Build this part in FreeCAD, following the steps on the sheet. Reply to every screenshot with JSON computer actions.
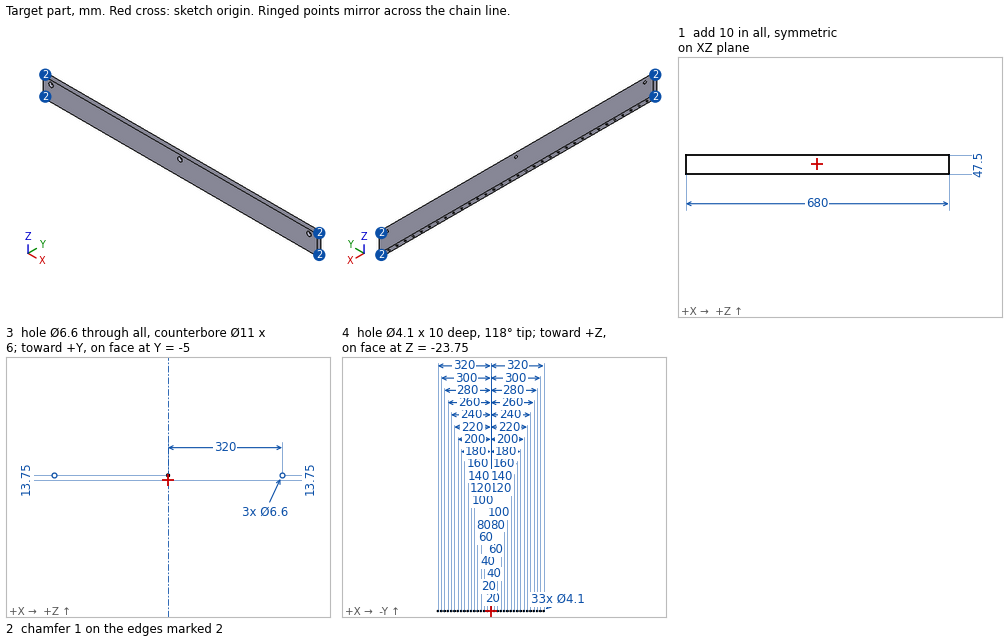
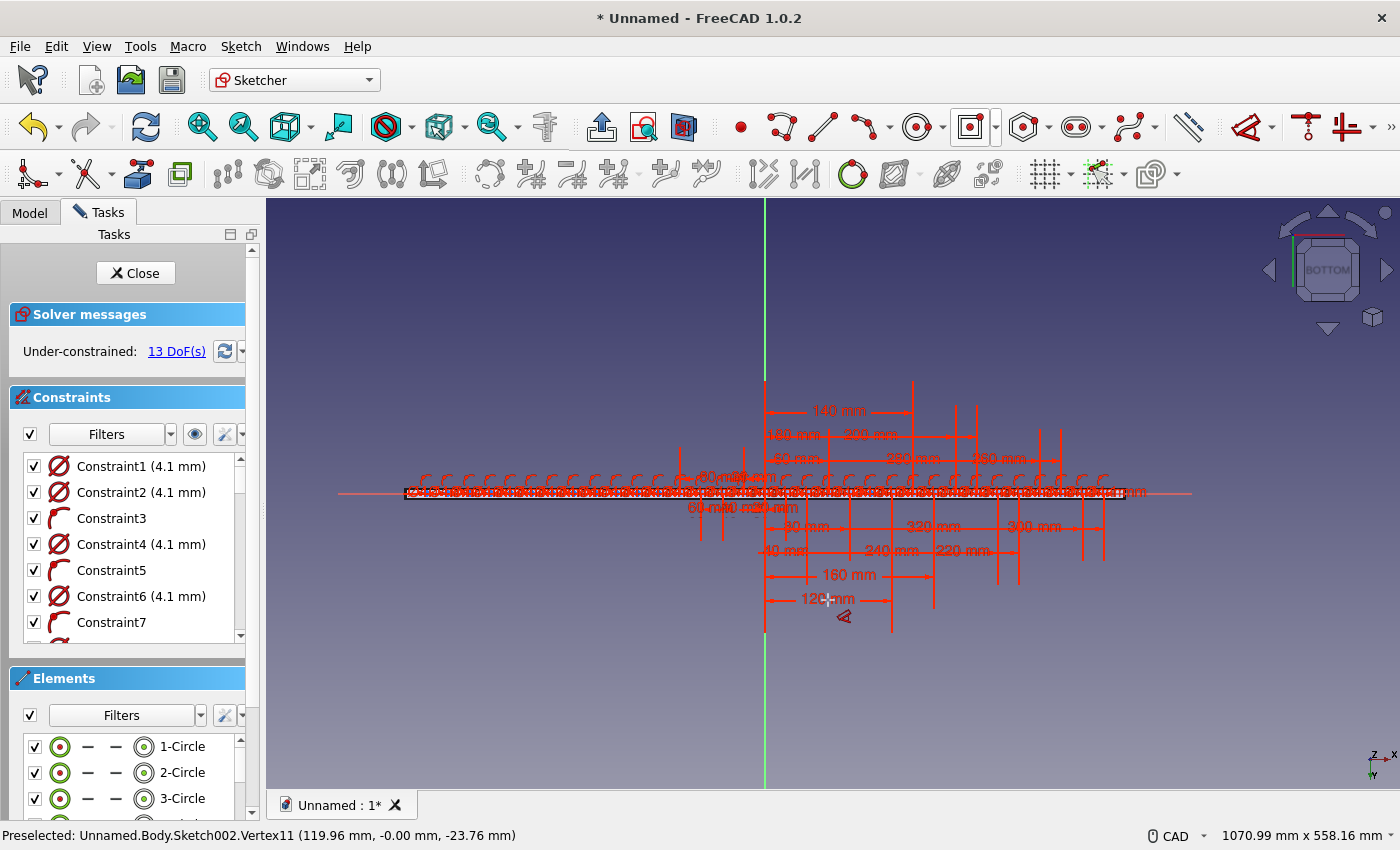
{"action": "left_click", "coordinate": [871, 494]}
{"action": "left_click", "coordinate": [818, 388]}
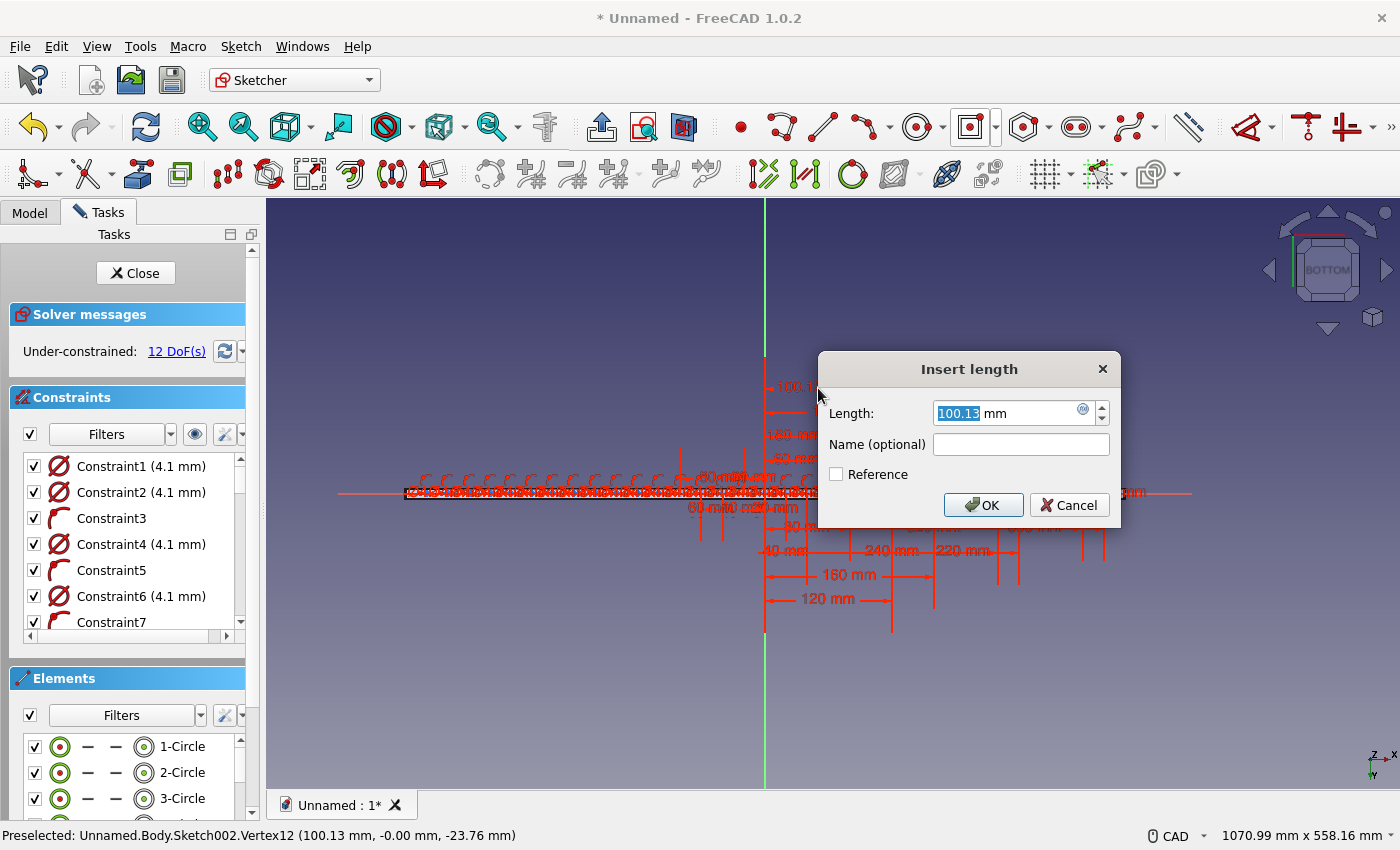
{"action": "type", "text": "100"}
{"action": "key", "text": "Return"}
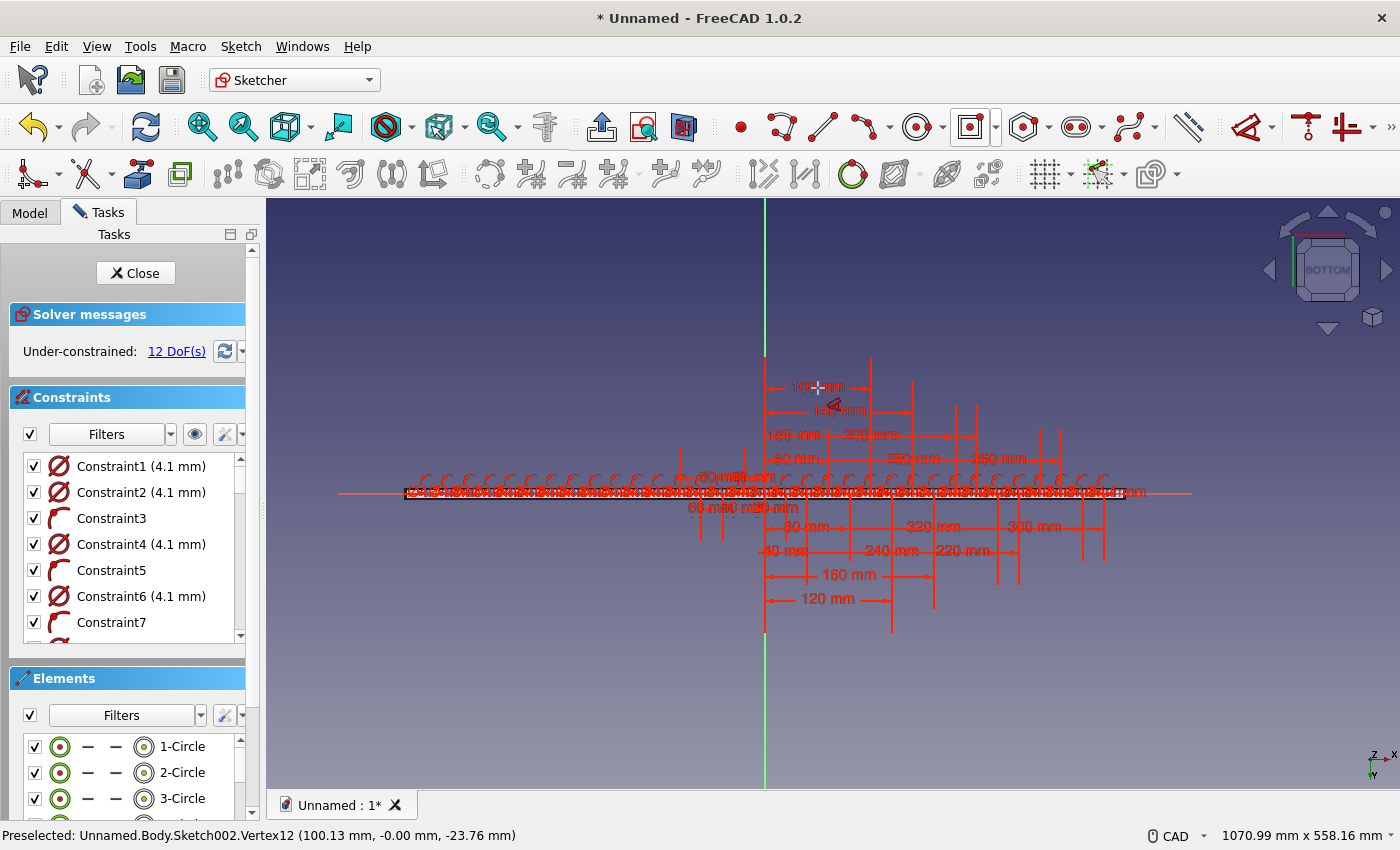
{"action": "left_click", "coordinate": [659, 494]}
{"action": "left_click", "coordinate": [712, 552]}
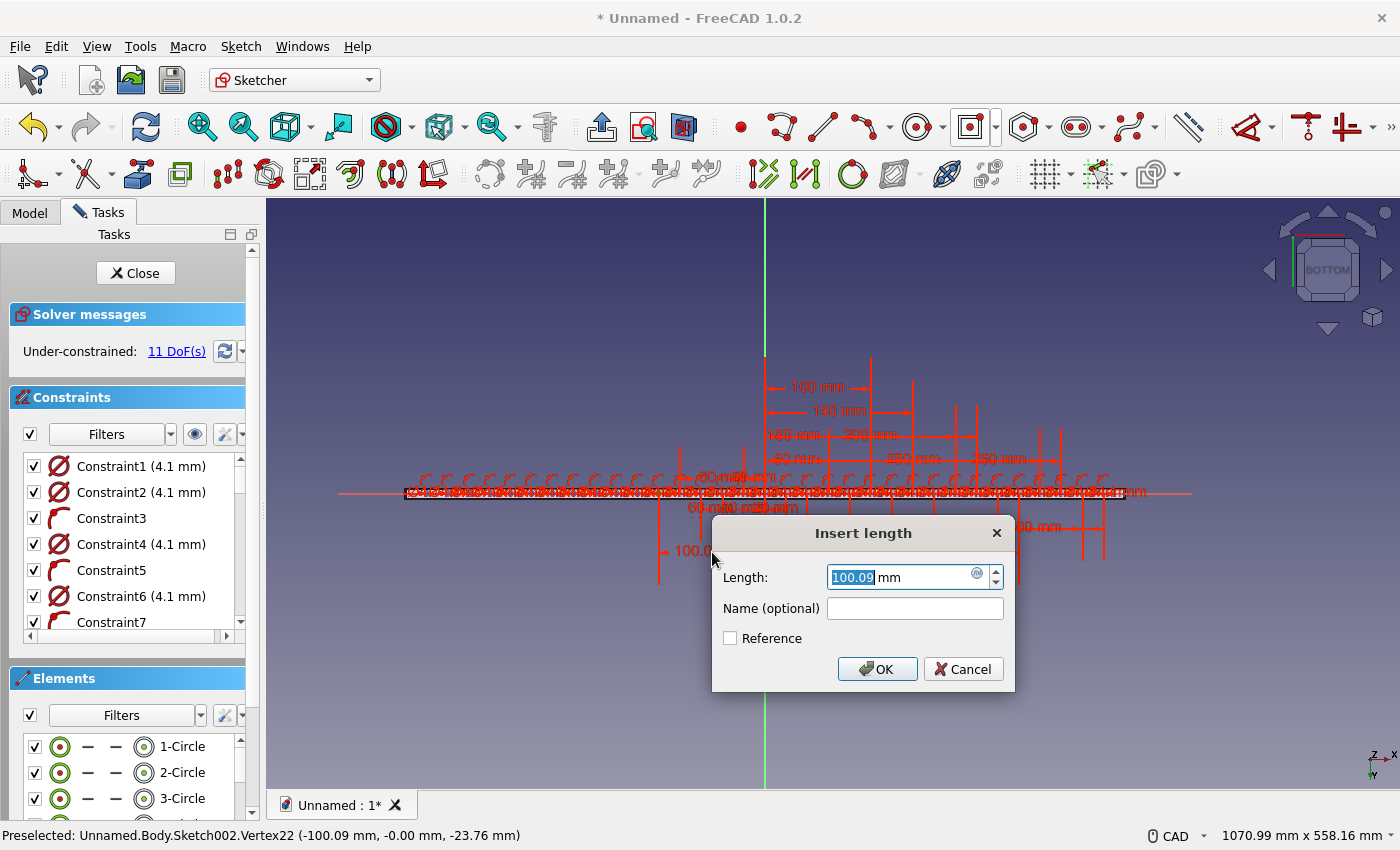
{"action": "type", "text": "100"}
{"action": "key", "text": "Return"}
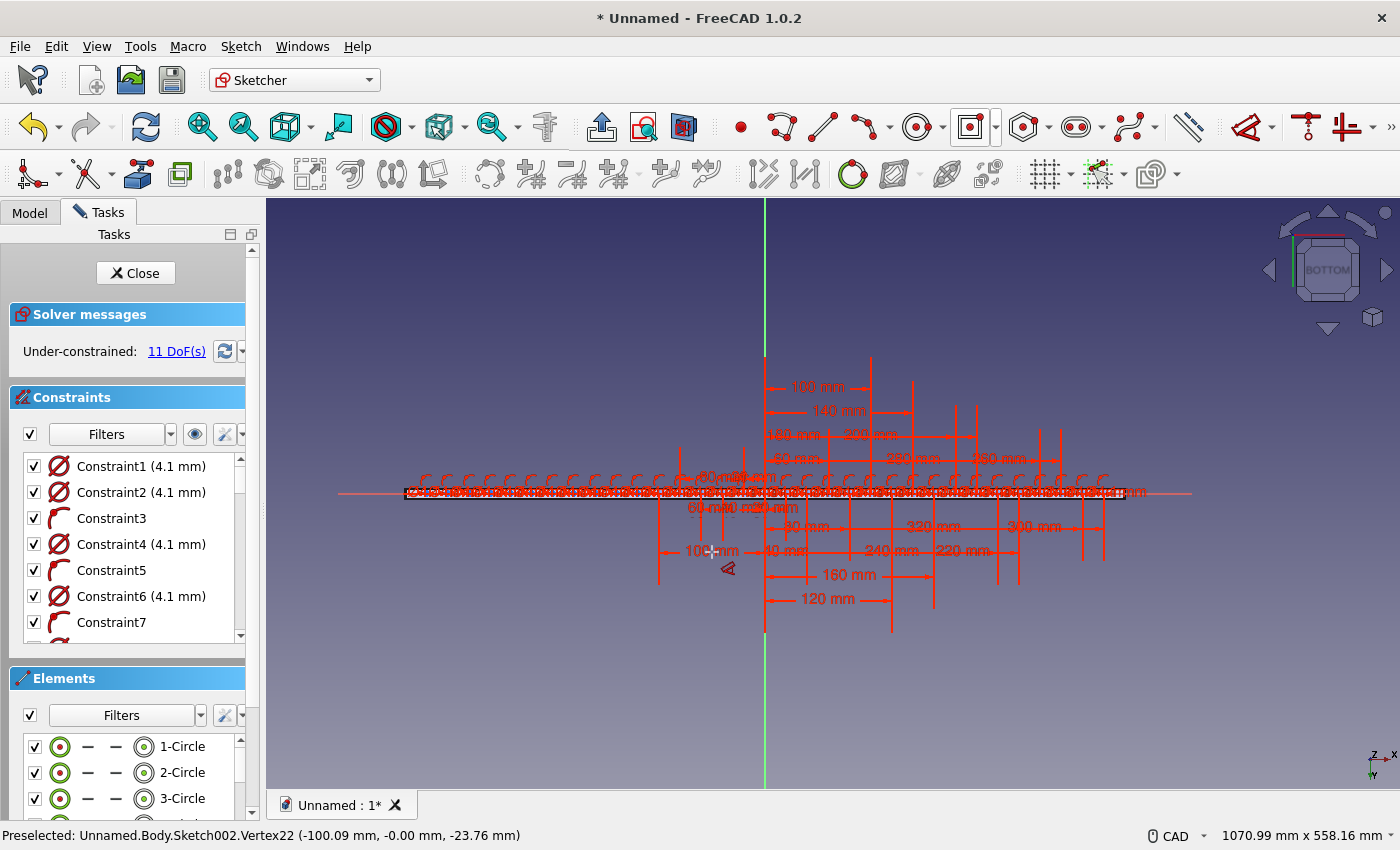
{"action": "left_click", "coordinate": [638, 494]}
{"action": "left_click", "coordinate": [701, 436]}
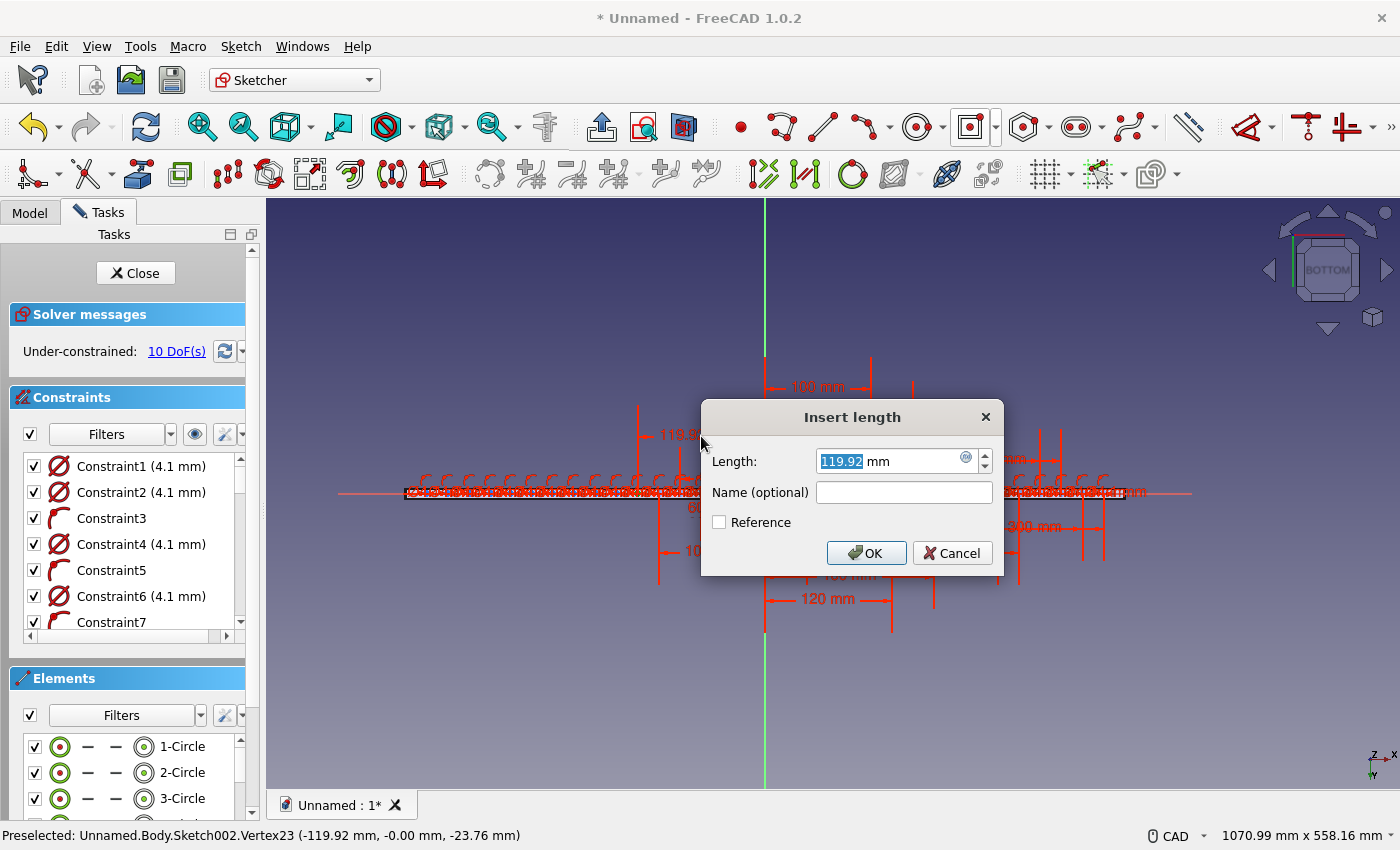
{"action": "type", "text": "120"}
{"action": "key", "text": "Return"}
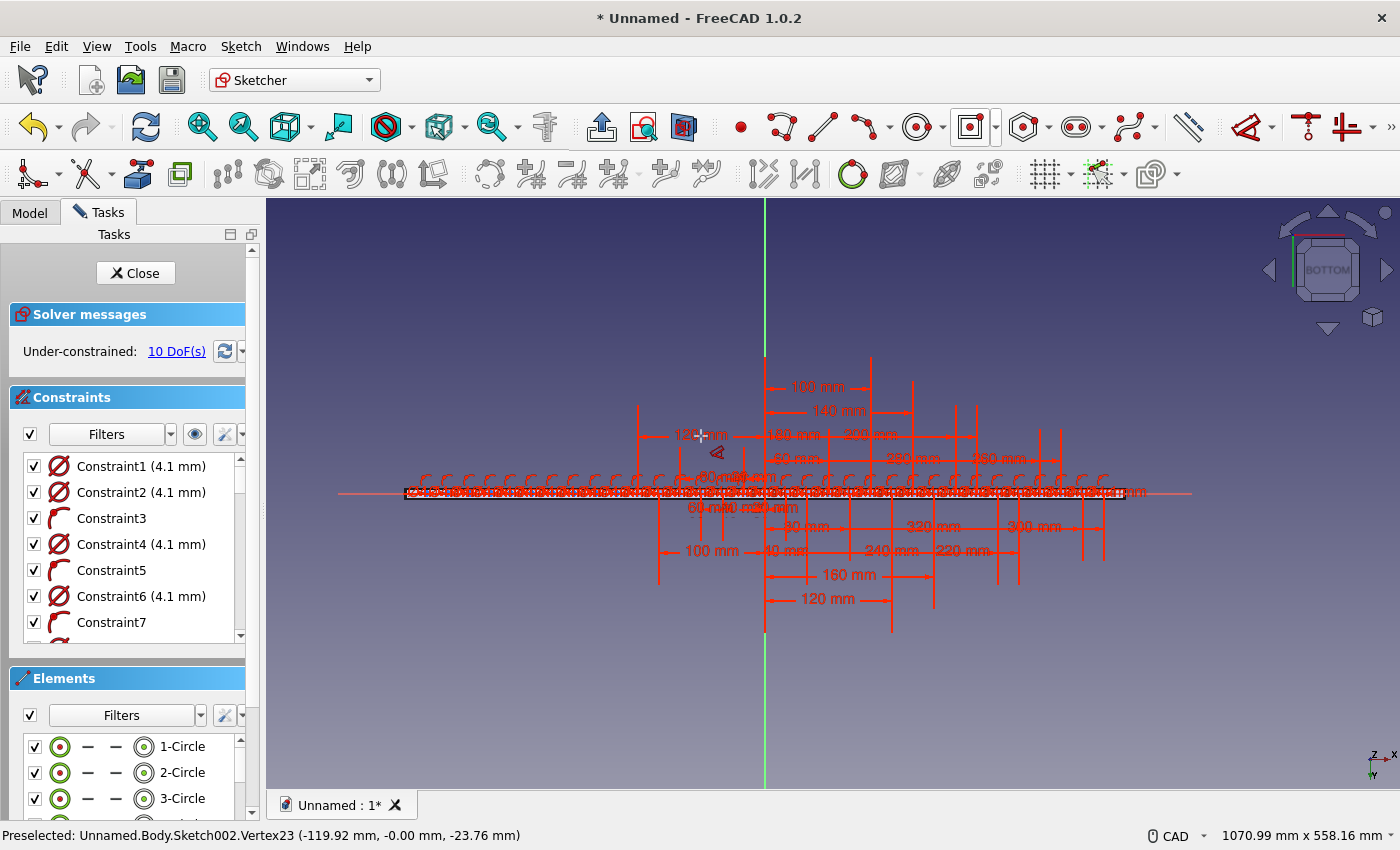
{"action": "left_click", "coordinate": [617, 494]}
{"action": "left_click", "coordinate": [639, 528]}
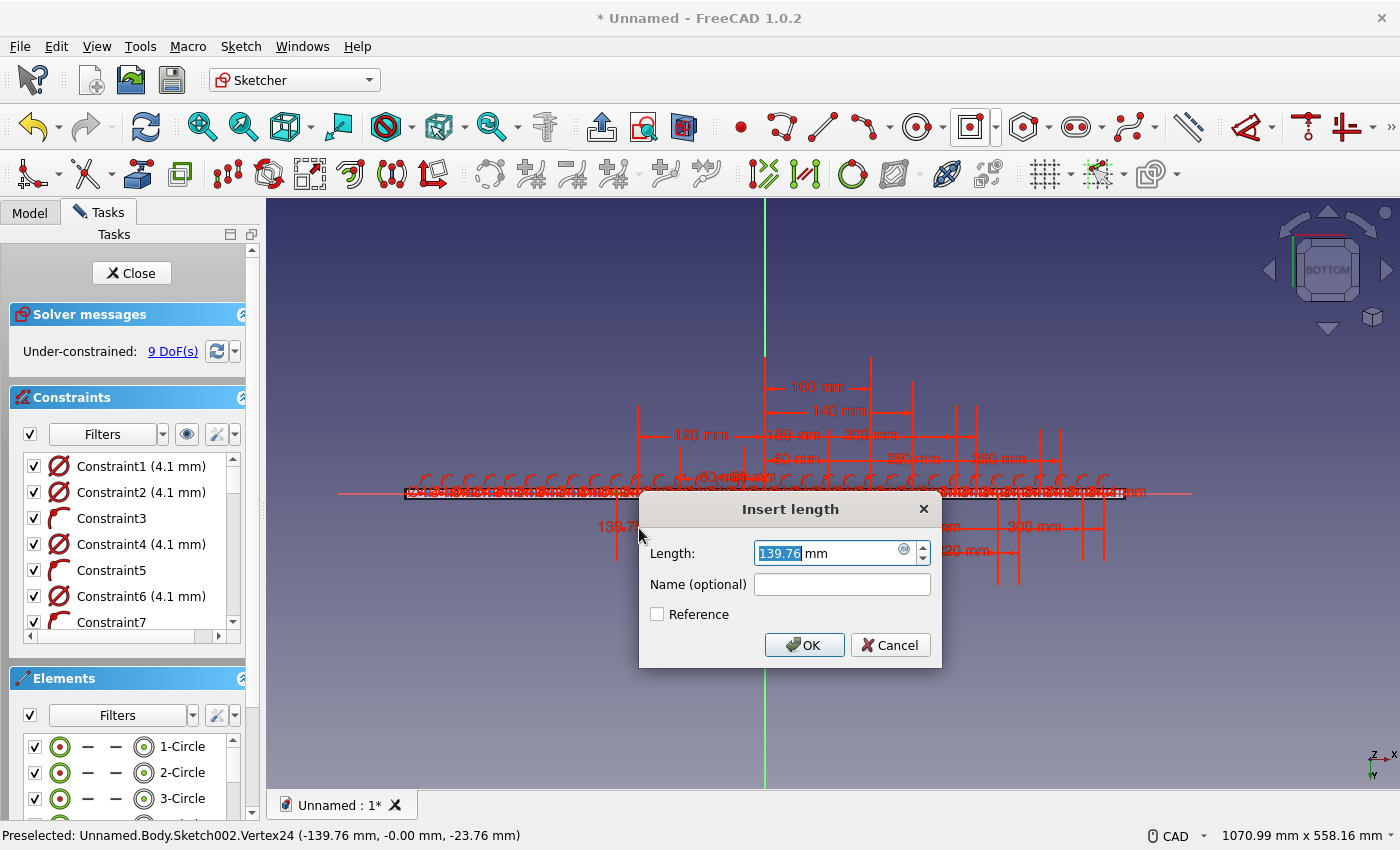
{"action": "type", "text": "140"}
{"action": "key", "text": "Return"}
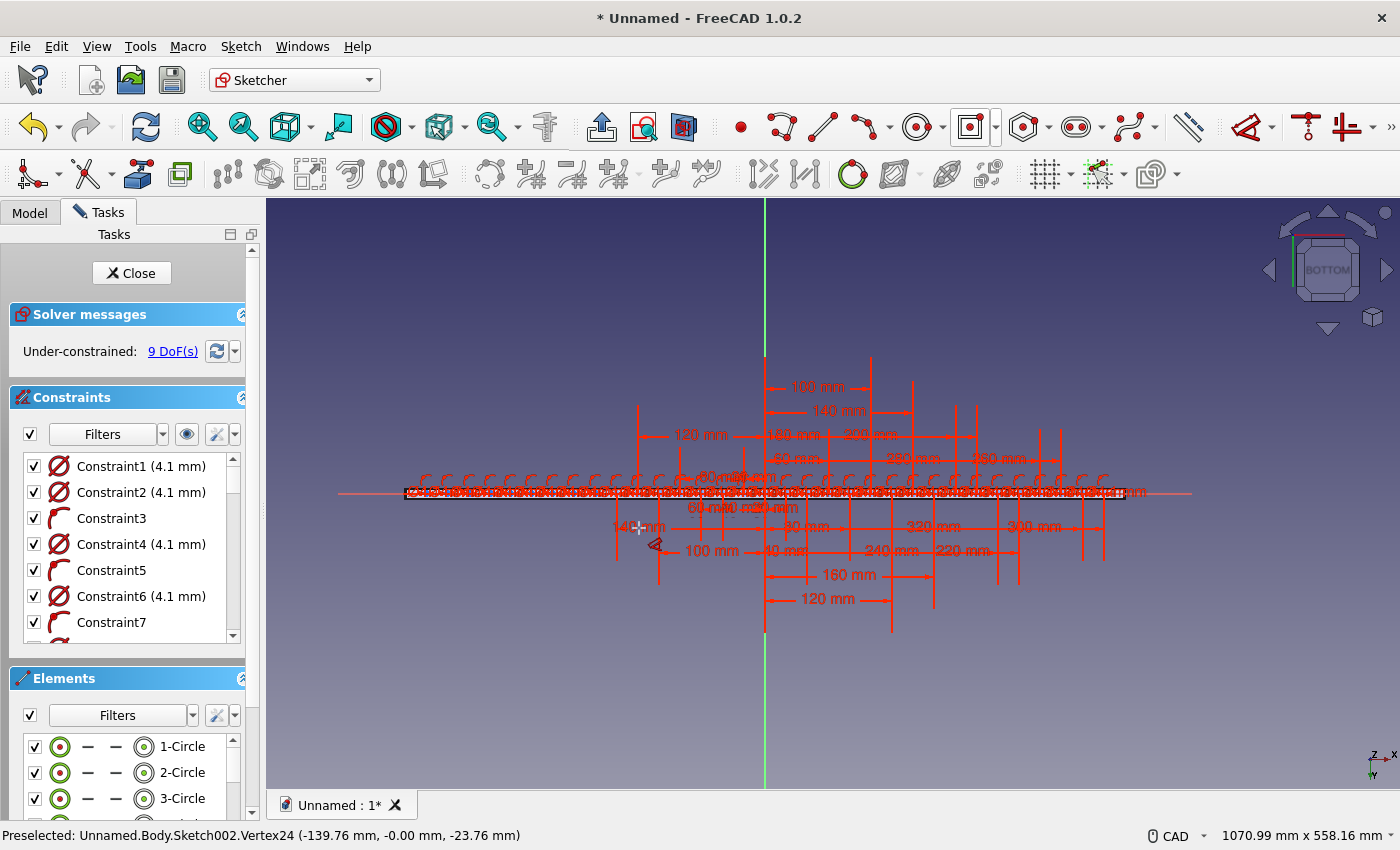
{"action": "left_click", "coordinate": [596, 494]}
{"action": "left_click", "coordinate": [642, 460]}